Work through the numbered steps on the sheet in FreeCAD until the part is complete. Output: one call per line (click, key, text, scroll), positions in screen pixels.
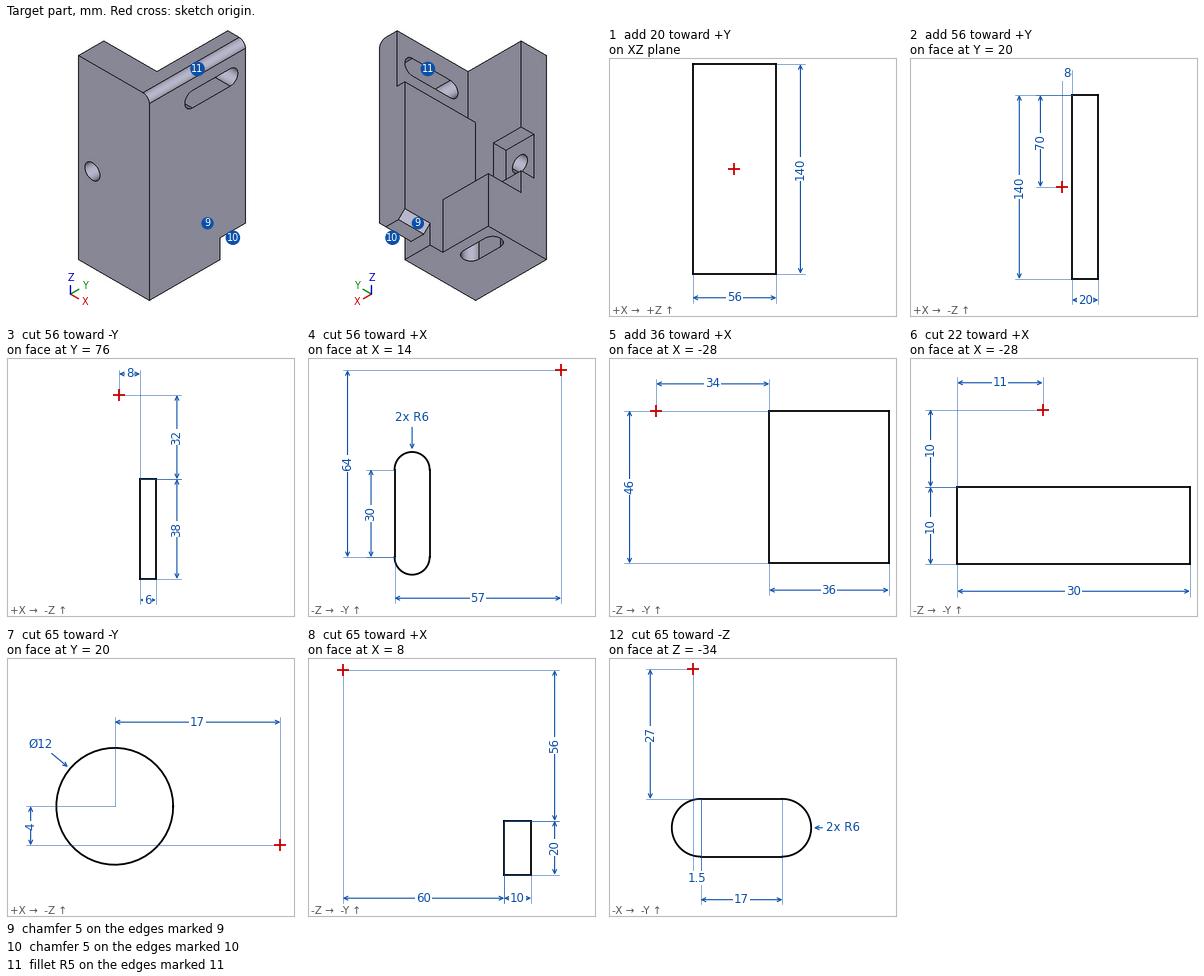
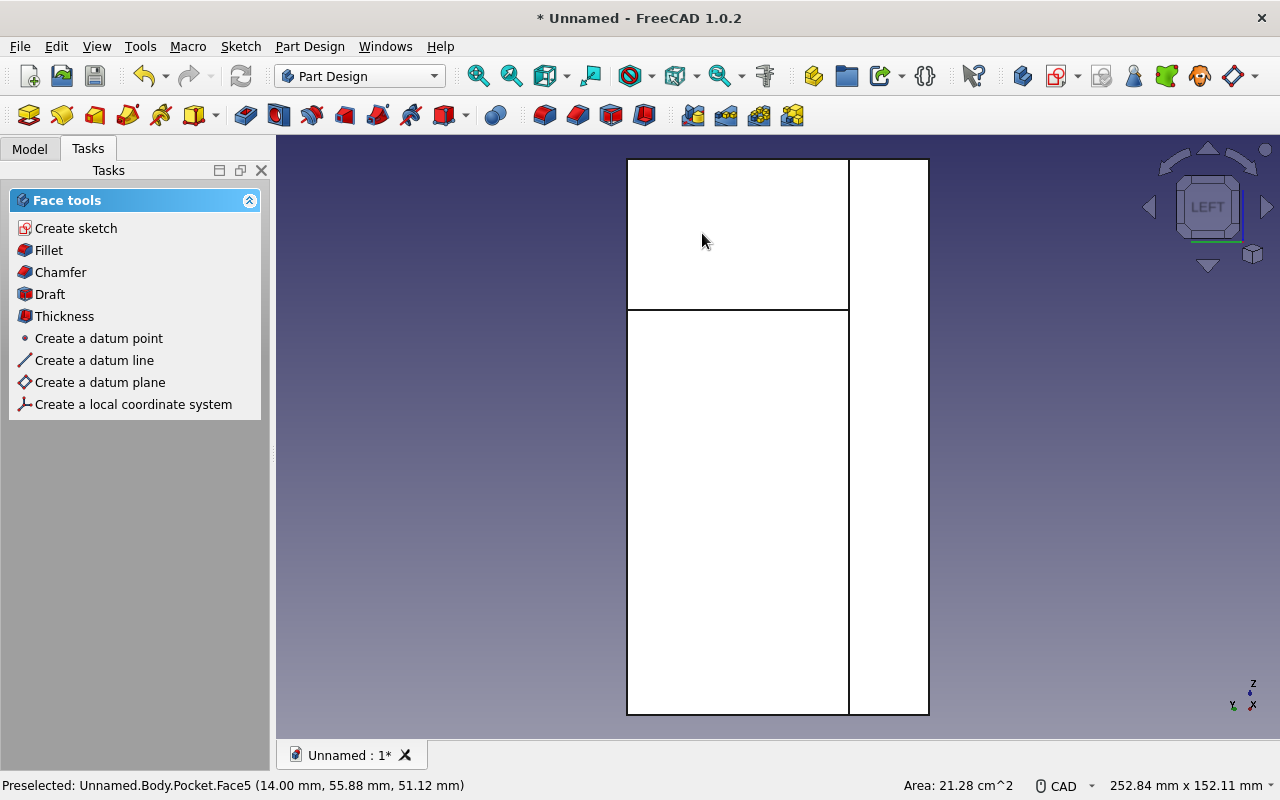
click(1056, 76)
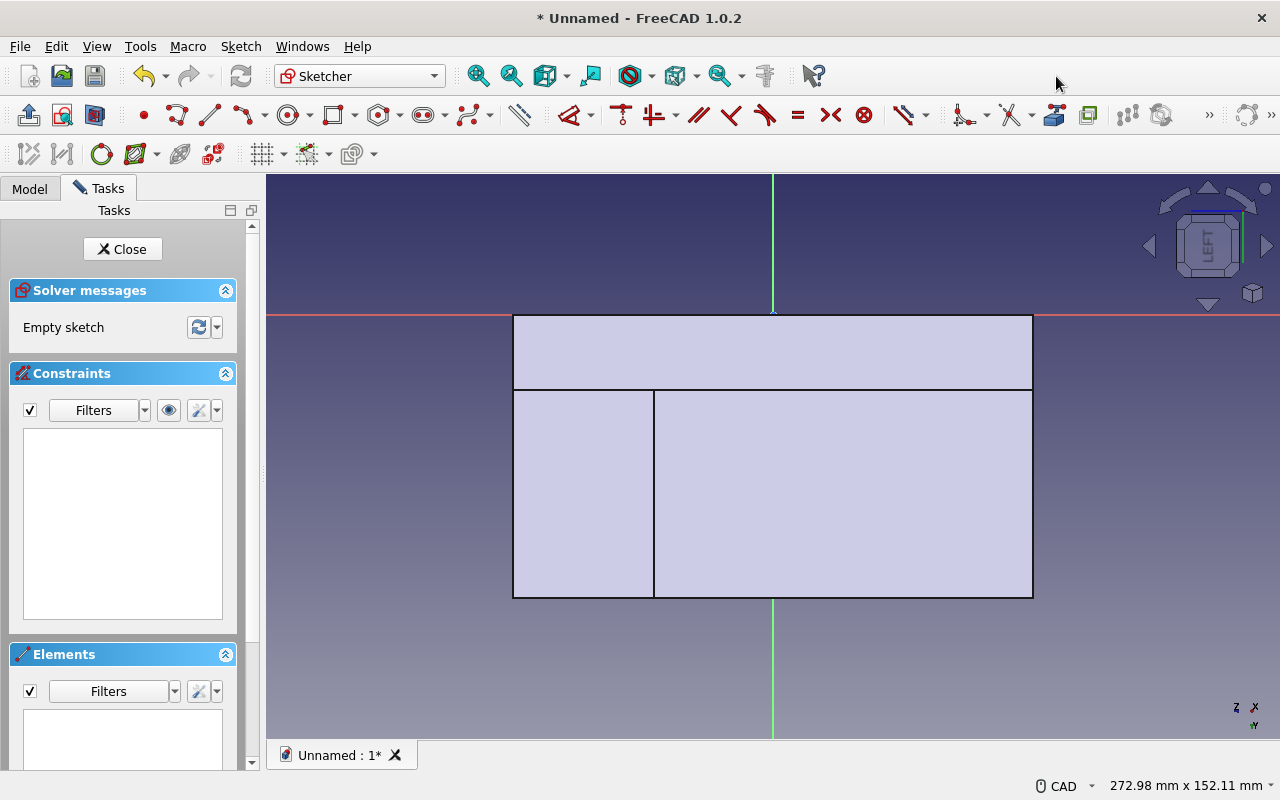
click(95, 116)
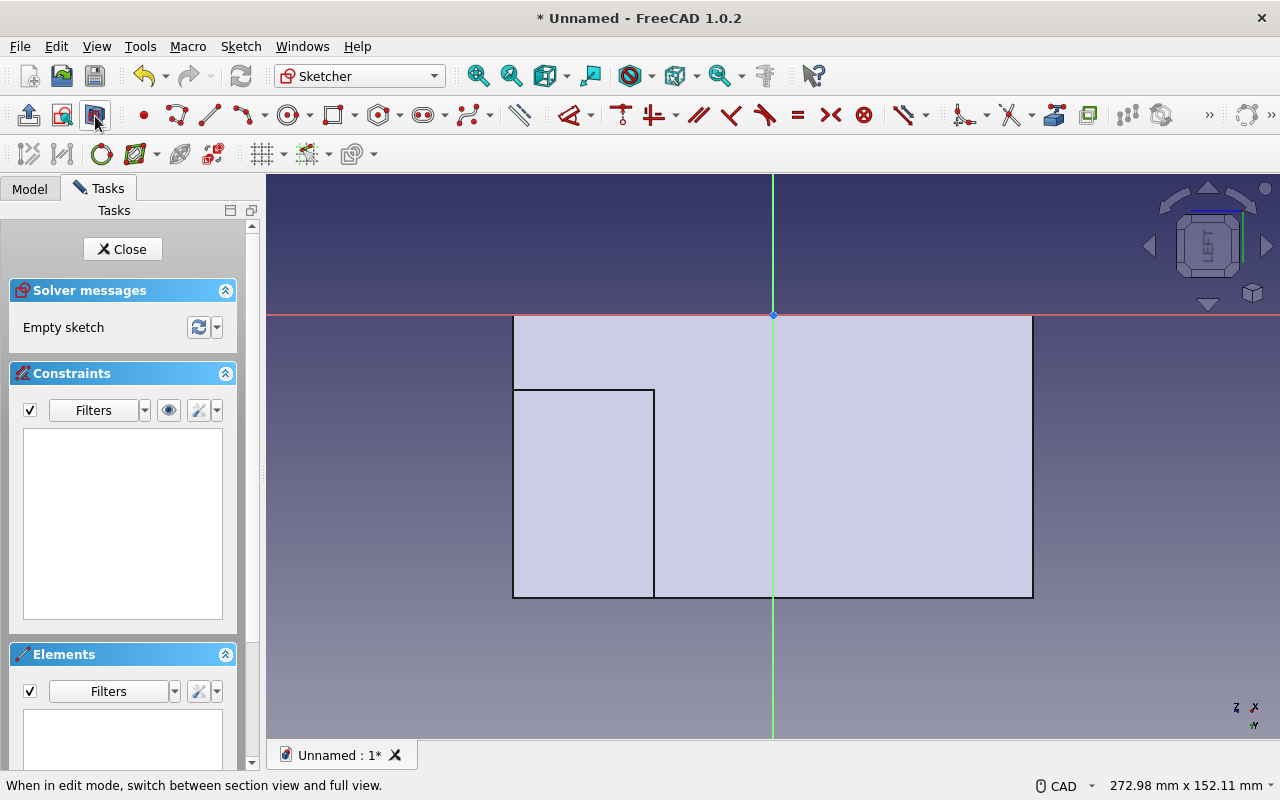
scroll(591, 423, up, 2)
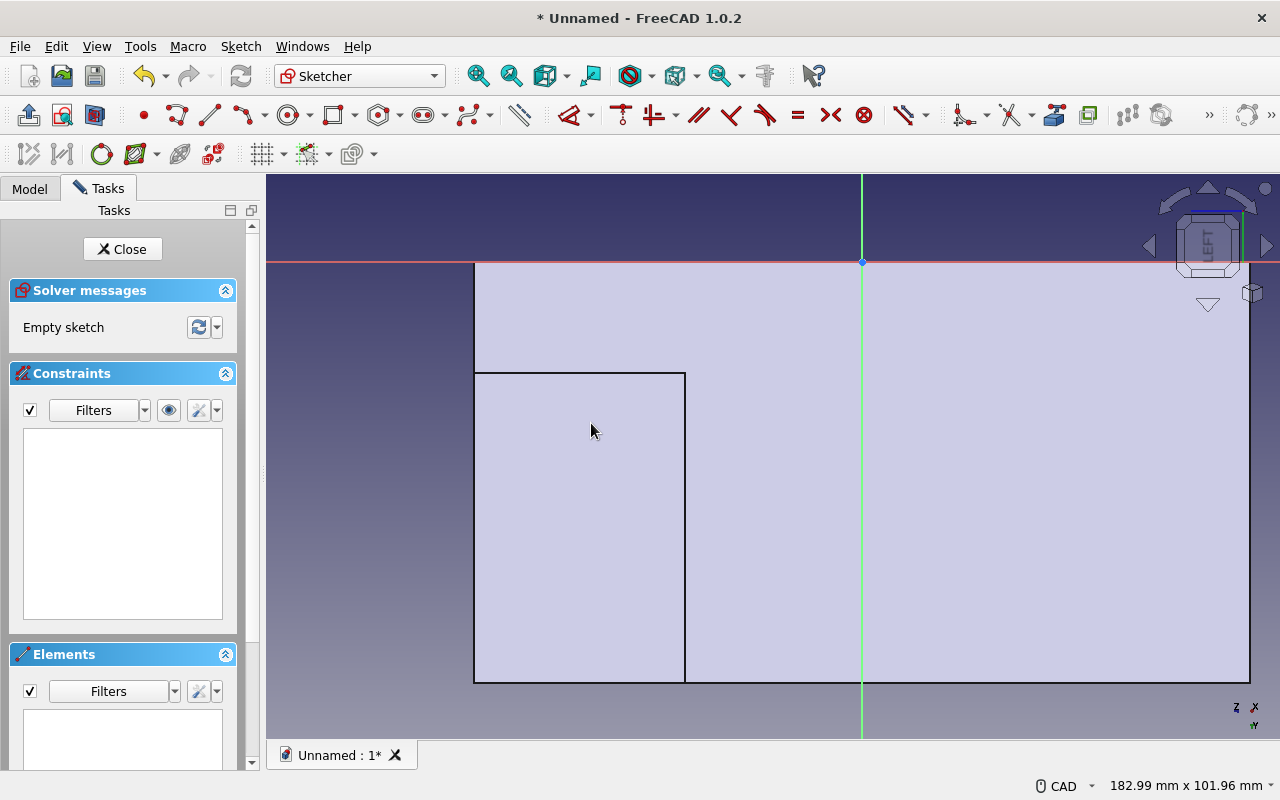
click(422, 116)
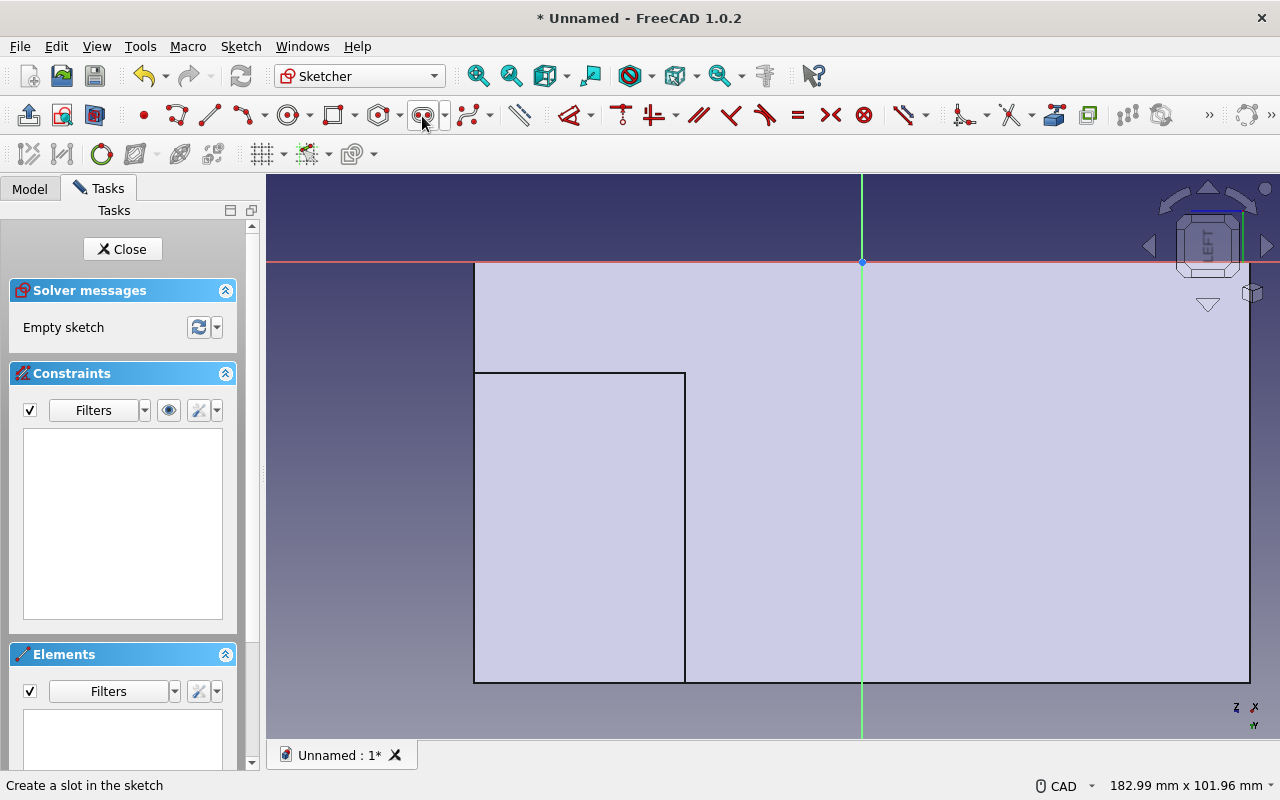
click(580, 617)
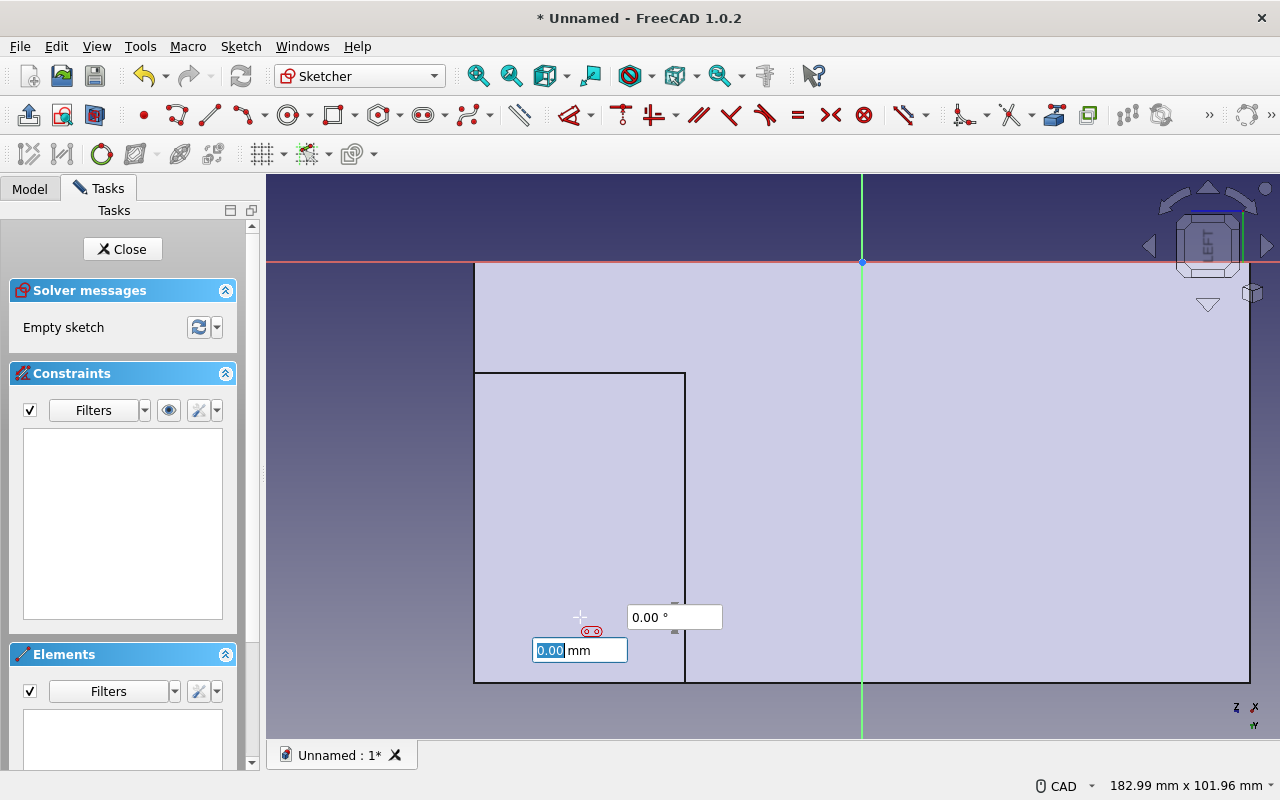
click(580, 451)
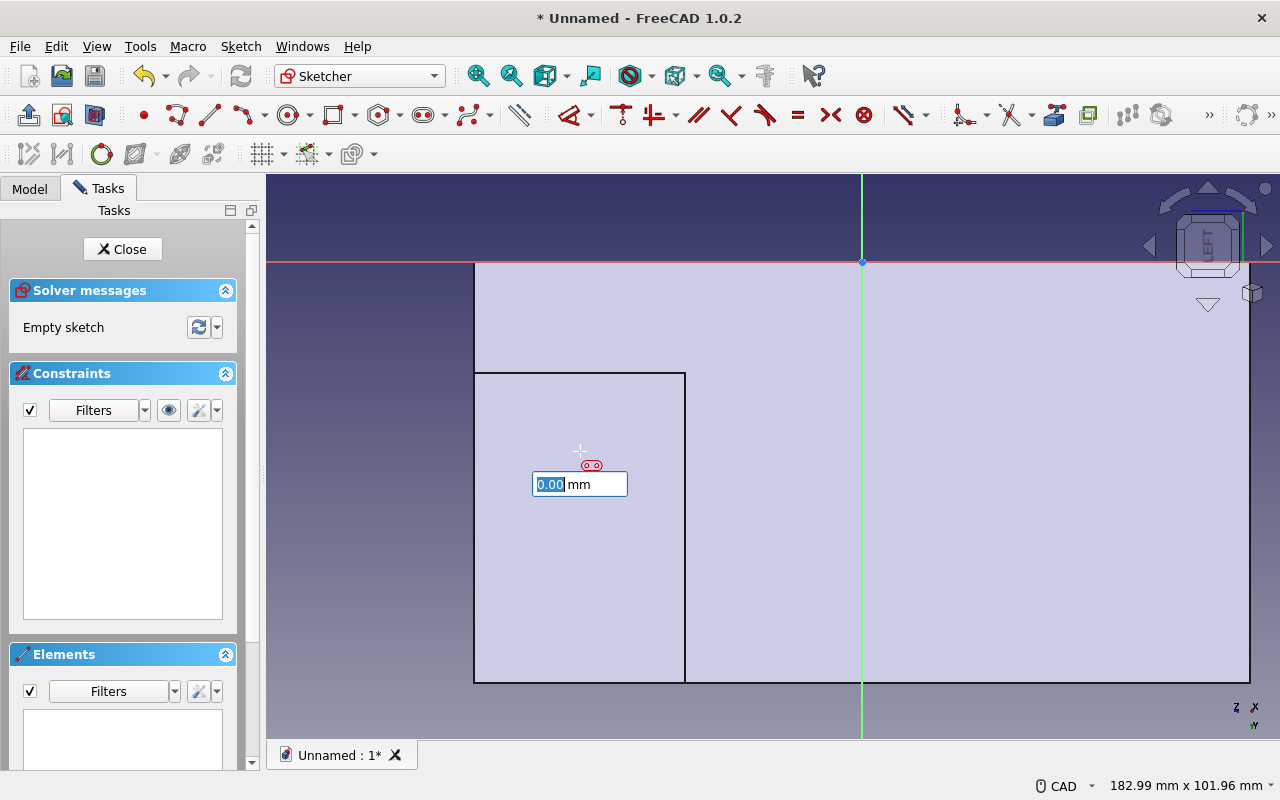
click(546, 534)
key(Escape)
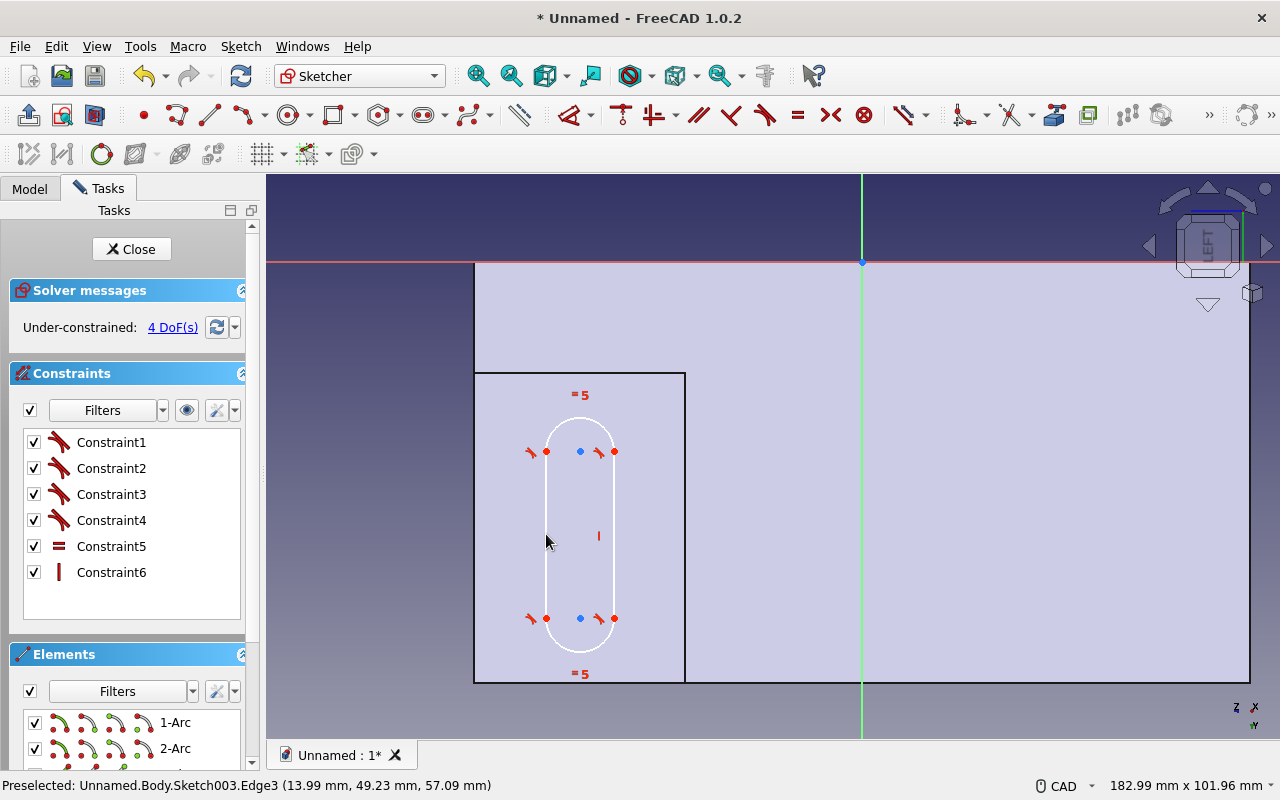
click(568, 116)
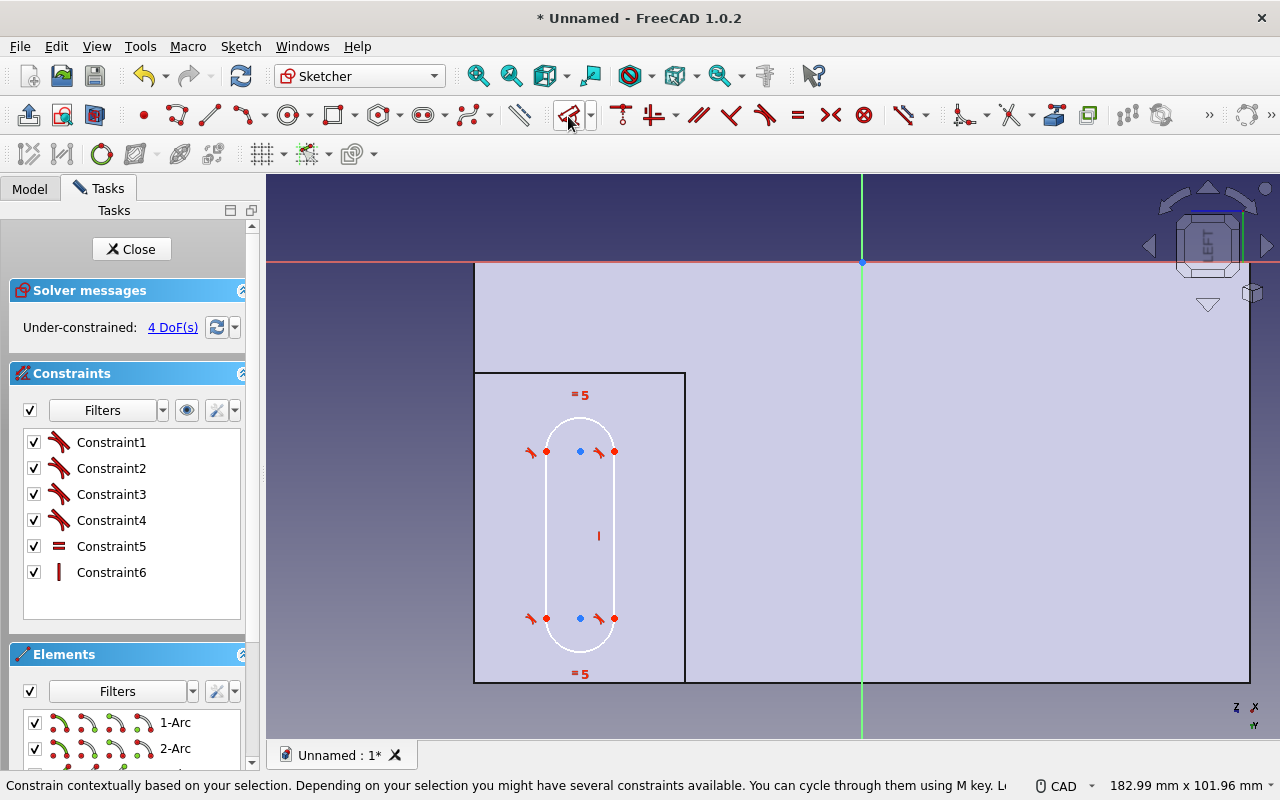
click(560, 646)
click(541, 672)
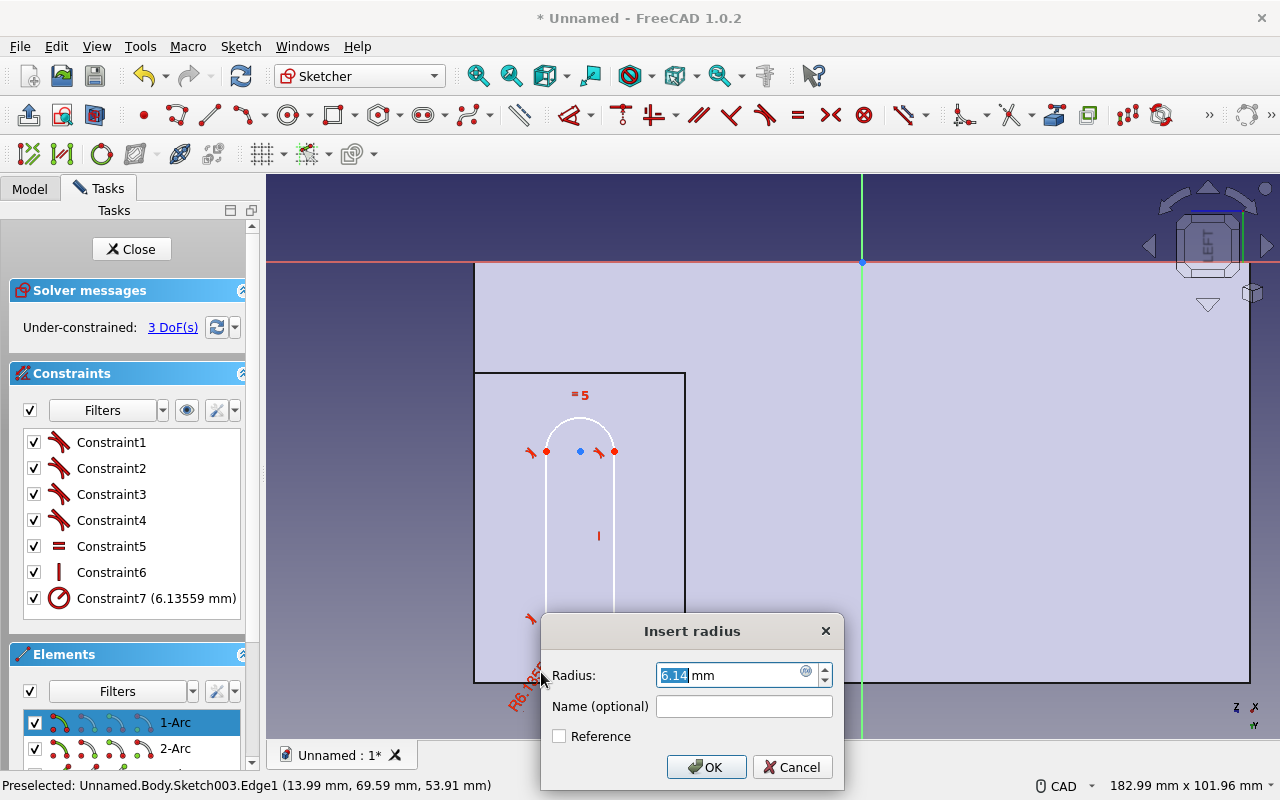
text(6)
key(Return)